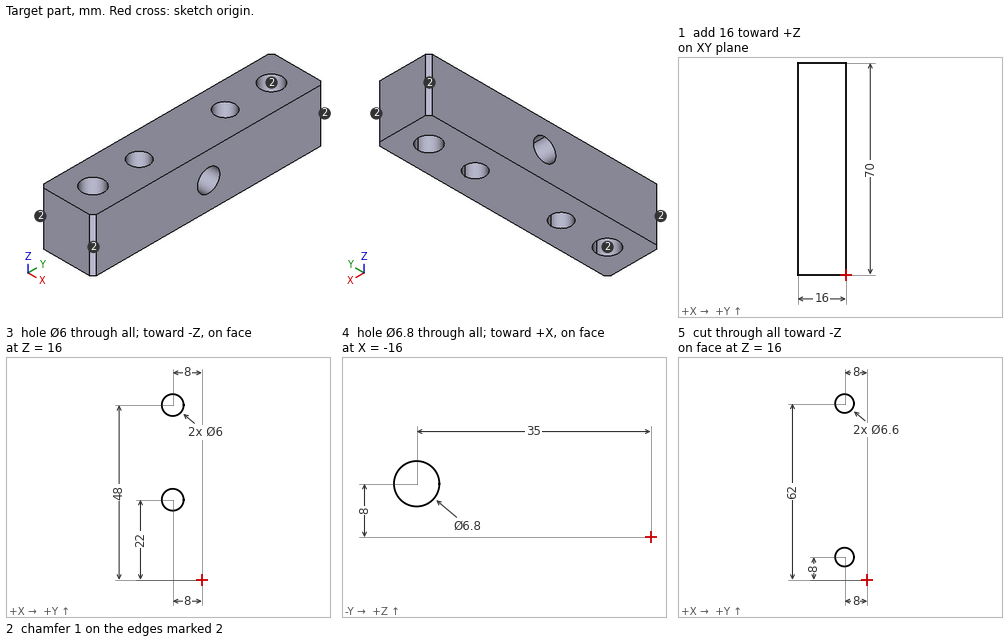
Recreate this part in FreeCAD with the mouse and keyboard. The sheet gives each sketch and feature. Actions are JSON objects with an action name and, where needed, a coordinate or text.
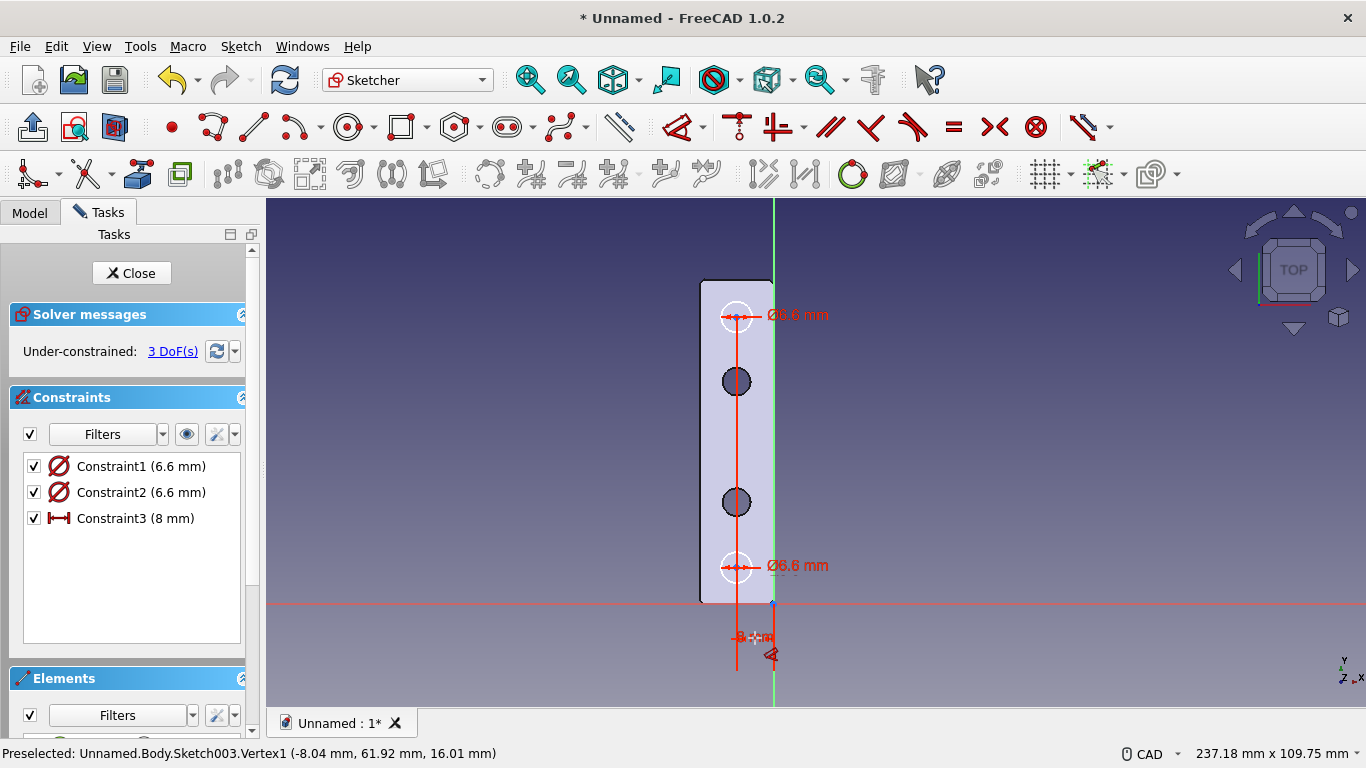
{"action": "left_click", "coordinate": [736, 568]}
{"action": "left_click", "coordinate": [755, 534]}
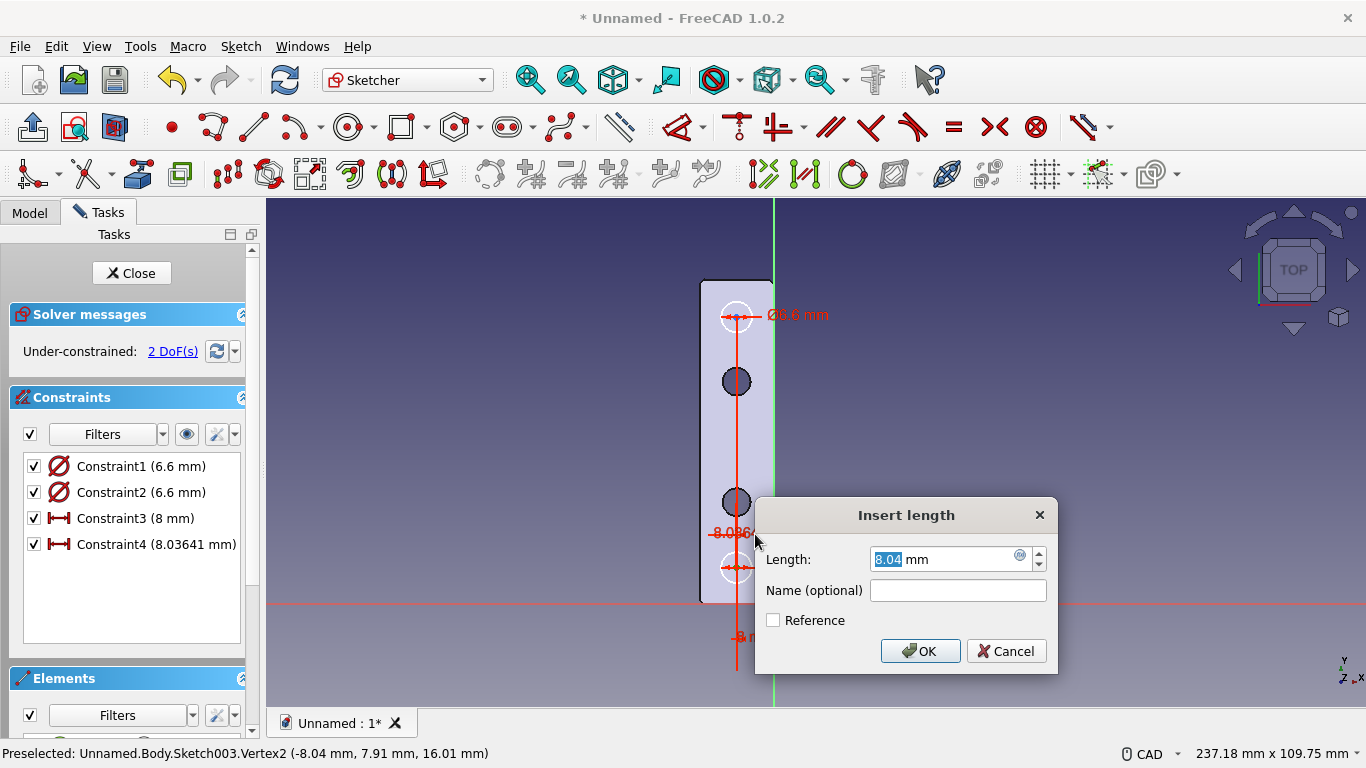
{"action": "type", "text": "8"}
{"action": "key", "text": "Return"}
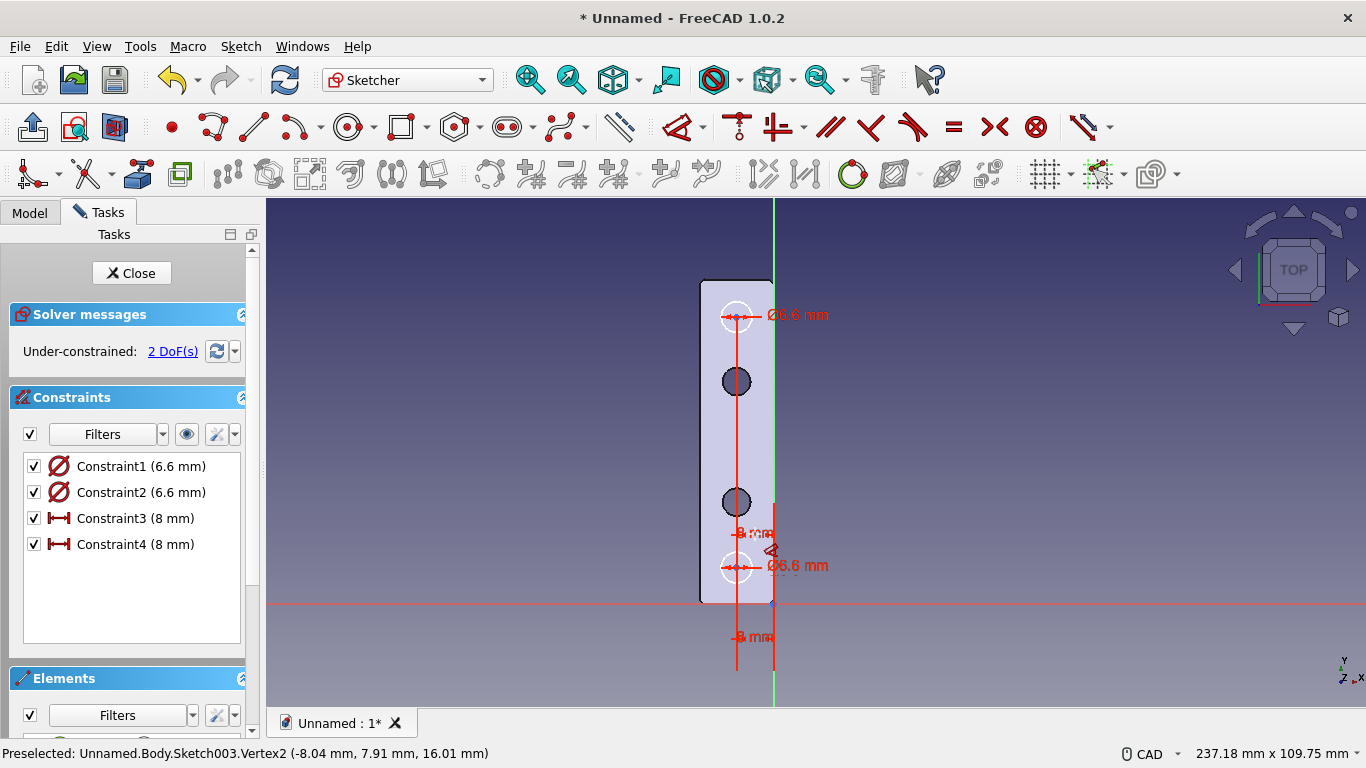
{"action": "left_click", "coordinate": [737, 568]}
{"action": "left_click", "coordinate": [808, 586]}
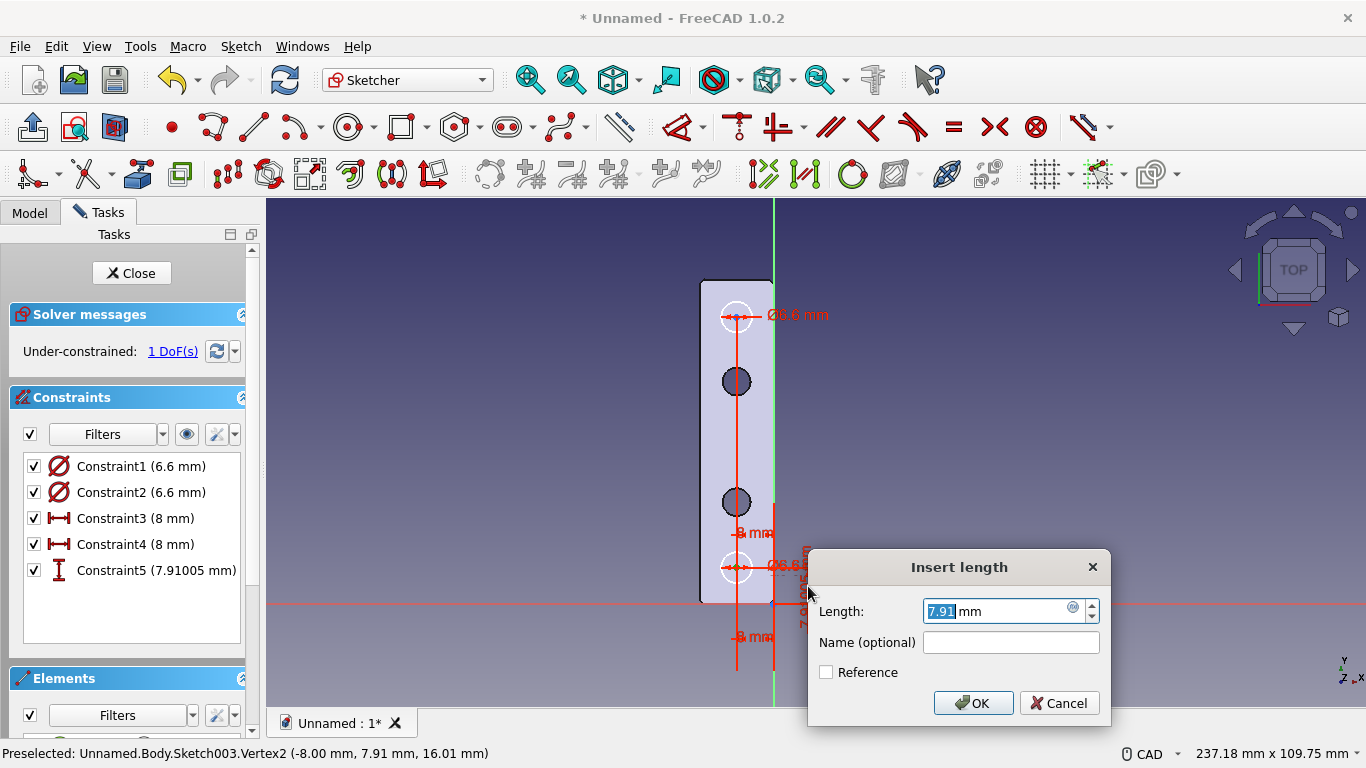
{"action": "type", "text": "8"}
{"action": "key", "text": "Return"}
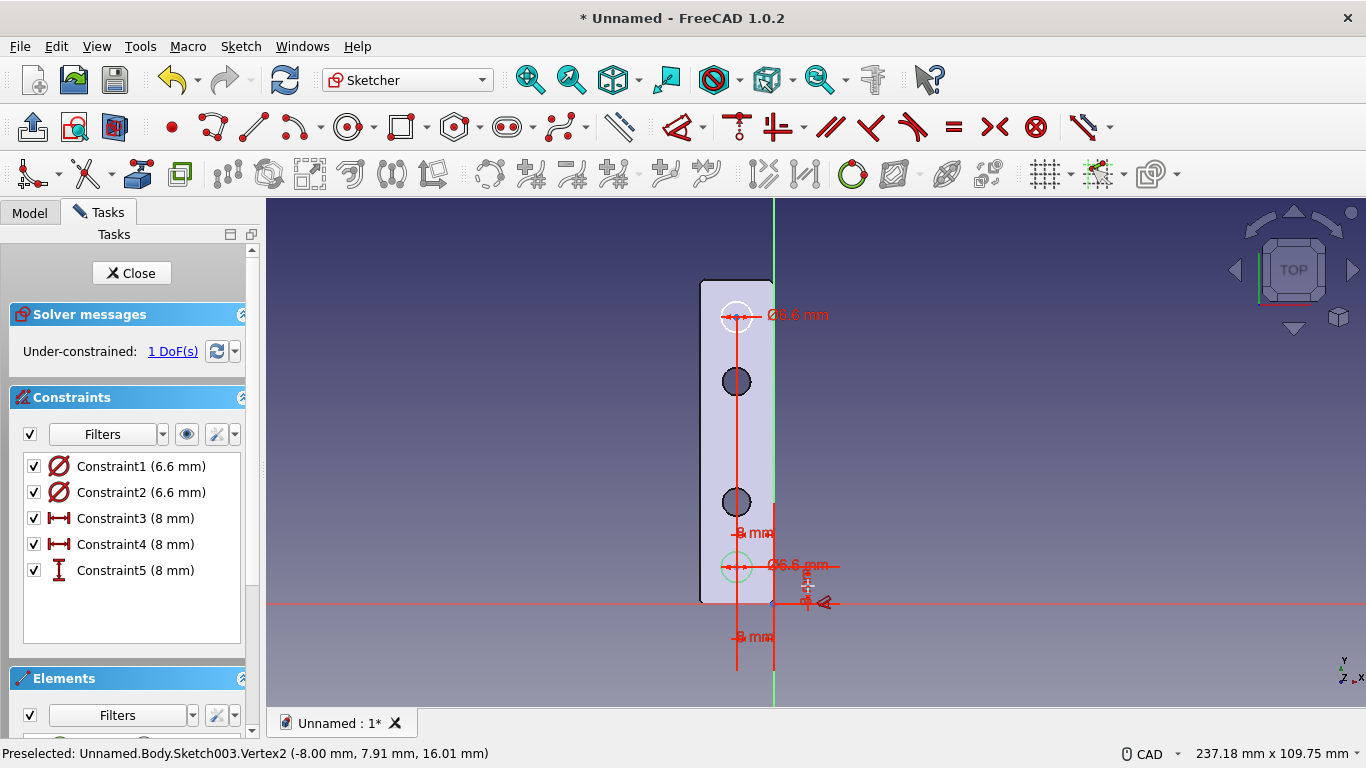
{"action": "left_click", "coordinate": [737, 317]}
{"action": "left_click", "coordinate": [808, 461]}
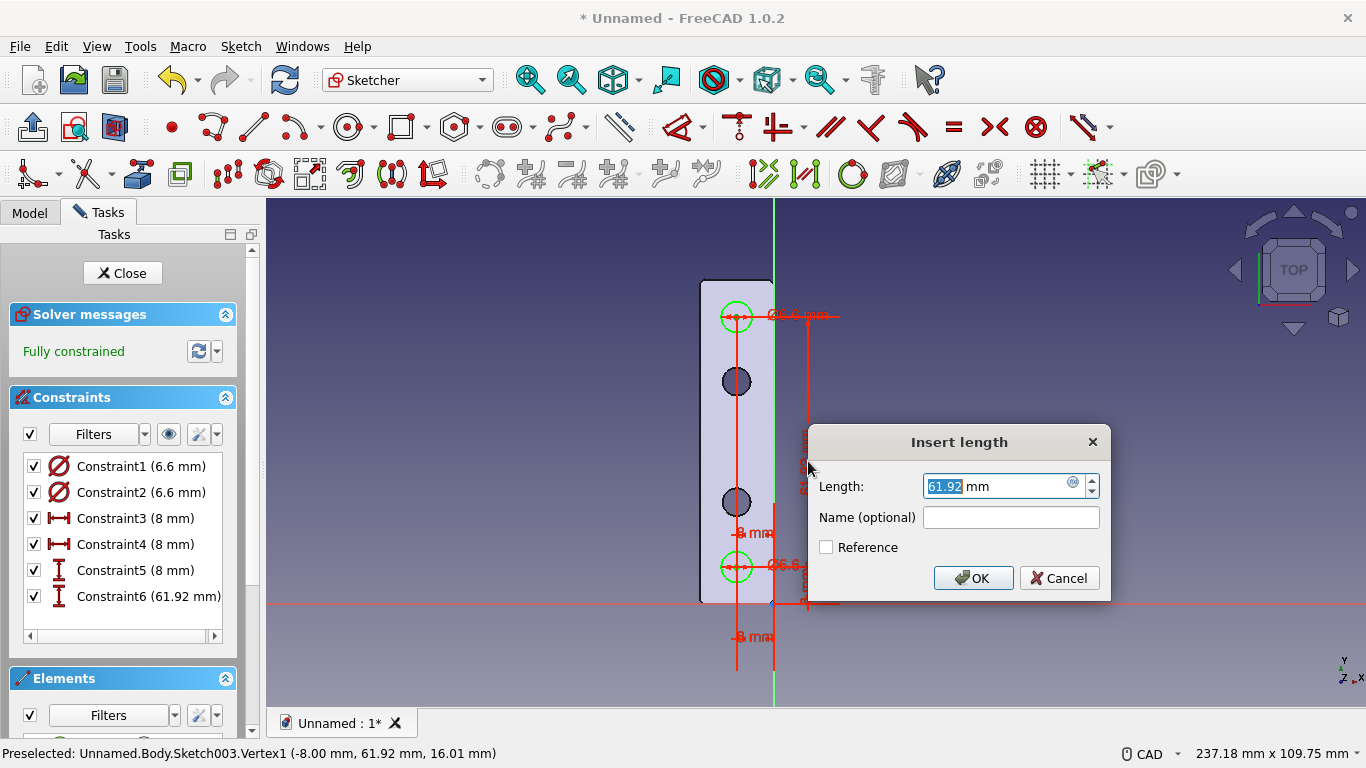
{"action": "type", "text": "62"}
{"action": "key", "text": "Return"}
{"action": "key", "text": "Escape"}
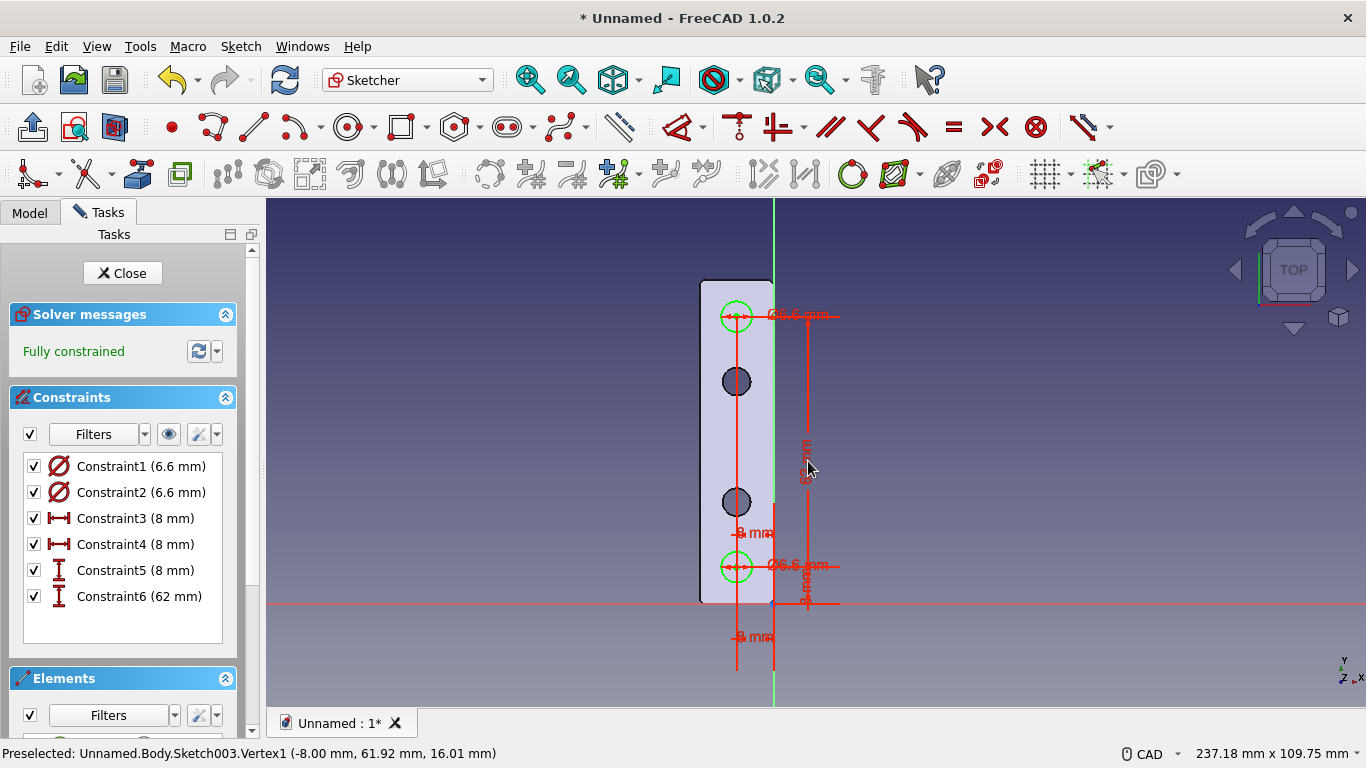
{"action": "left_click", "coordinate": [123, 273]}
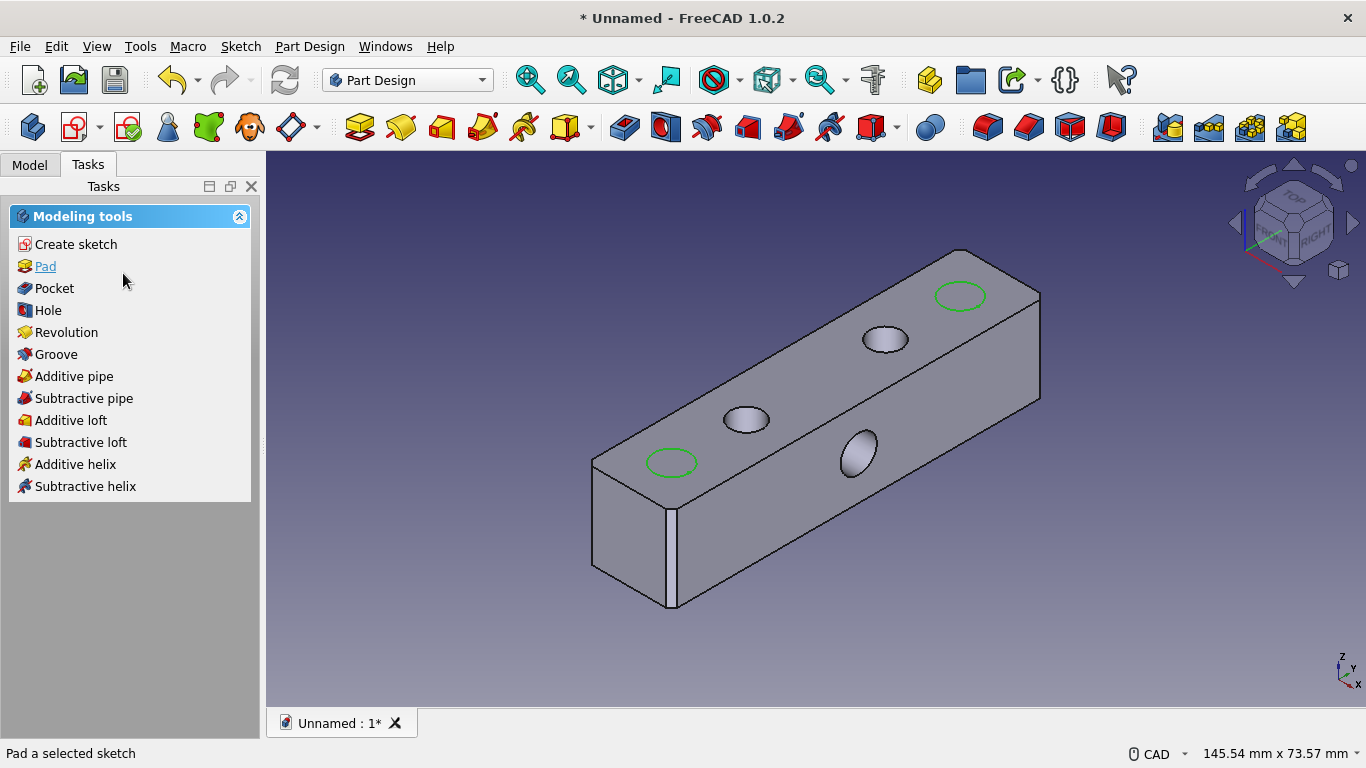
{"action": "left_click", "coordinate": [625, 128]}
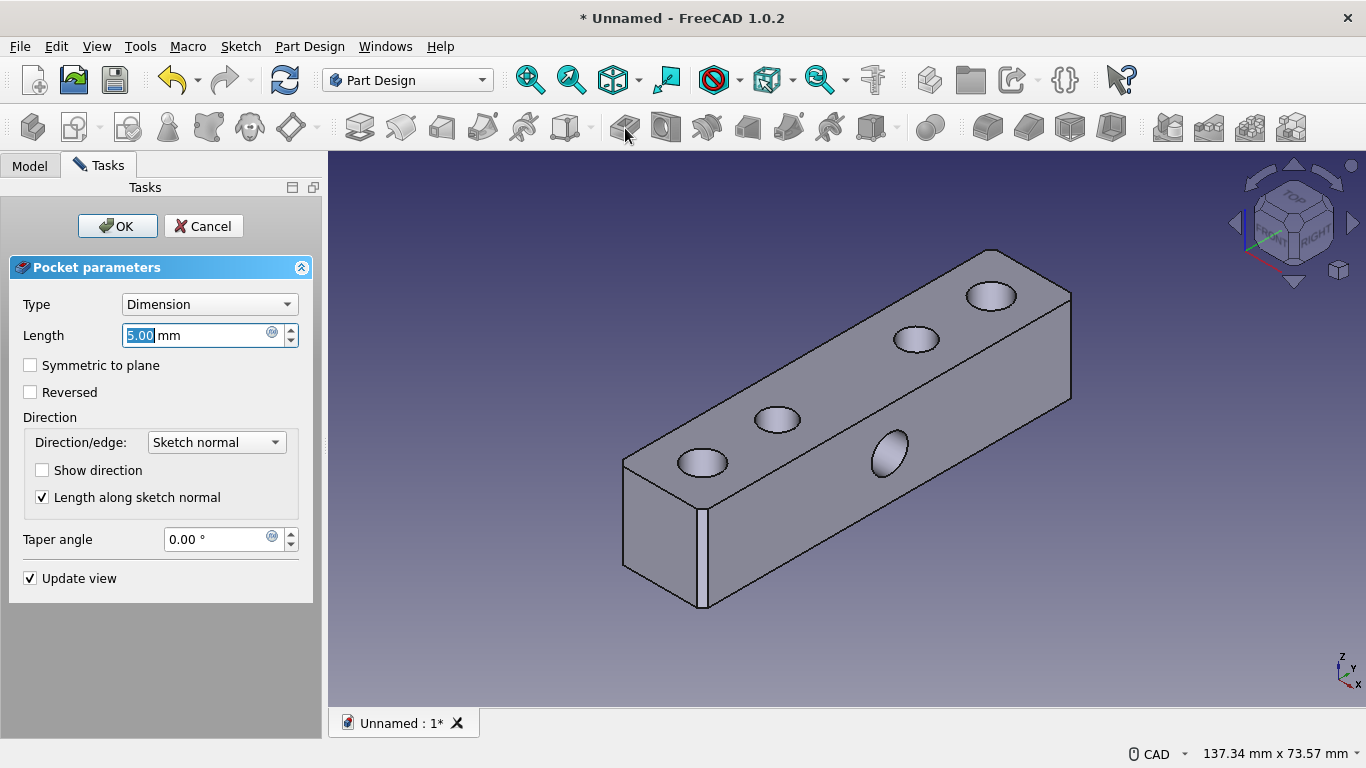
{"action": "left_click", "coordinate": [210, 304]}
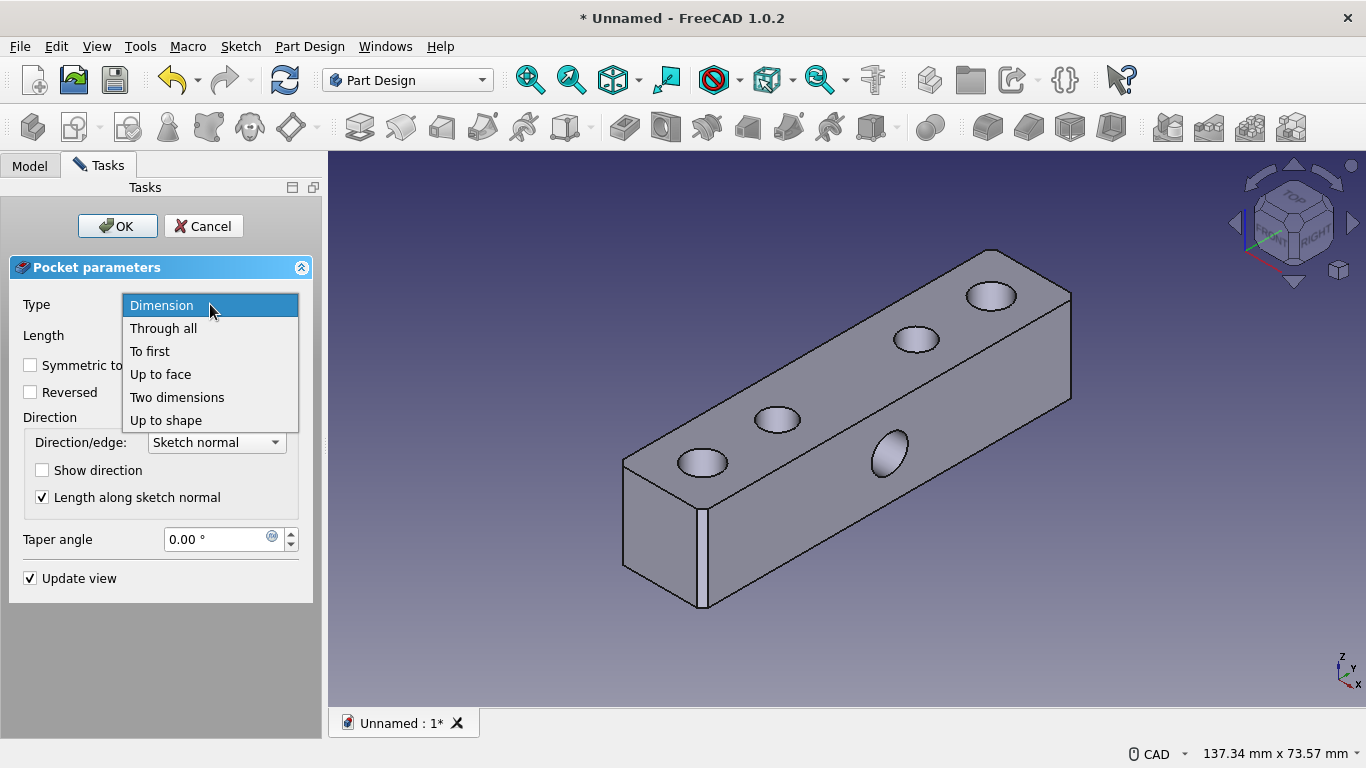
{"action": "left_click", "coordinate": [208, 328]}